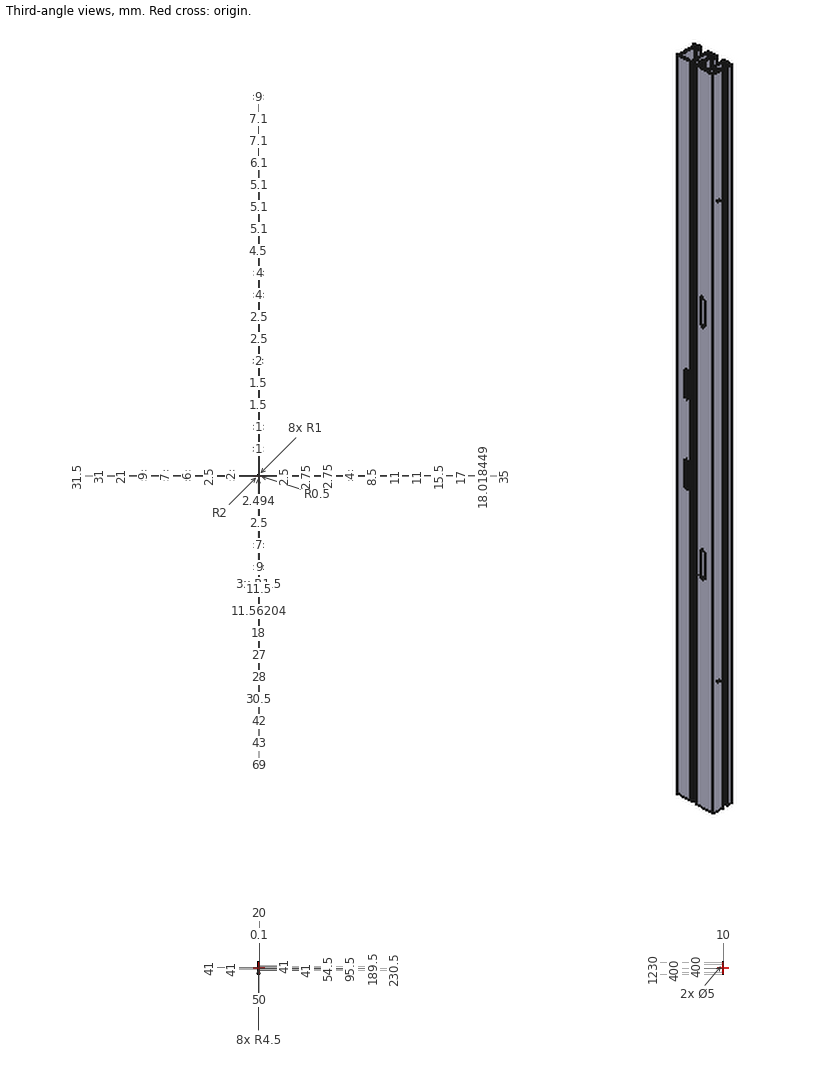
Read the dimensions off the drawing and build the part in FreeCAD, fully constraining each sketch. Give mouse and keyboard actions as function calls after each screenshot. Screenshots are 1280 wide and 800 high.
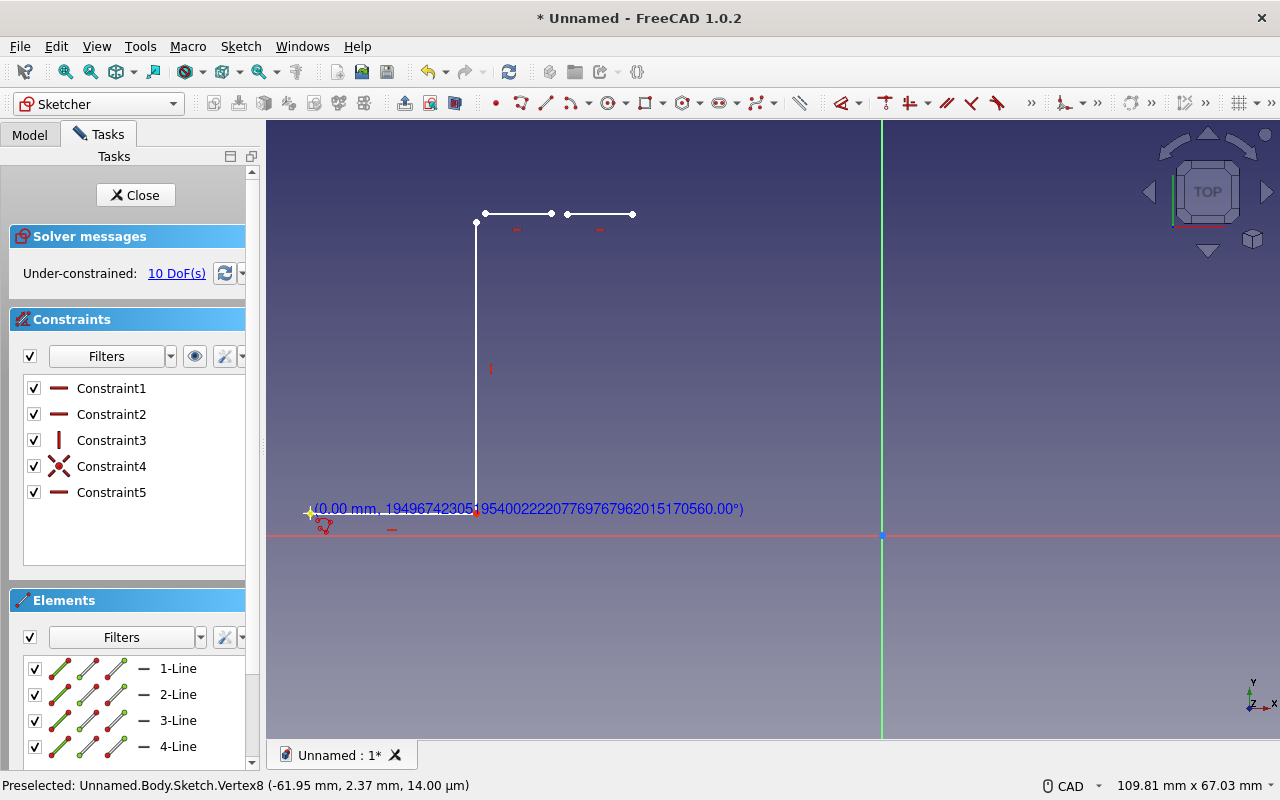
click(546, 104)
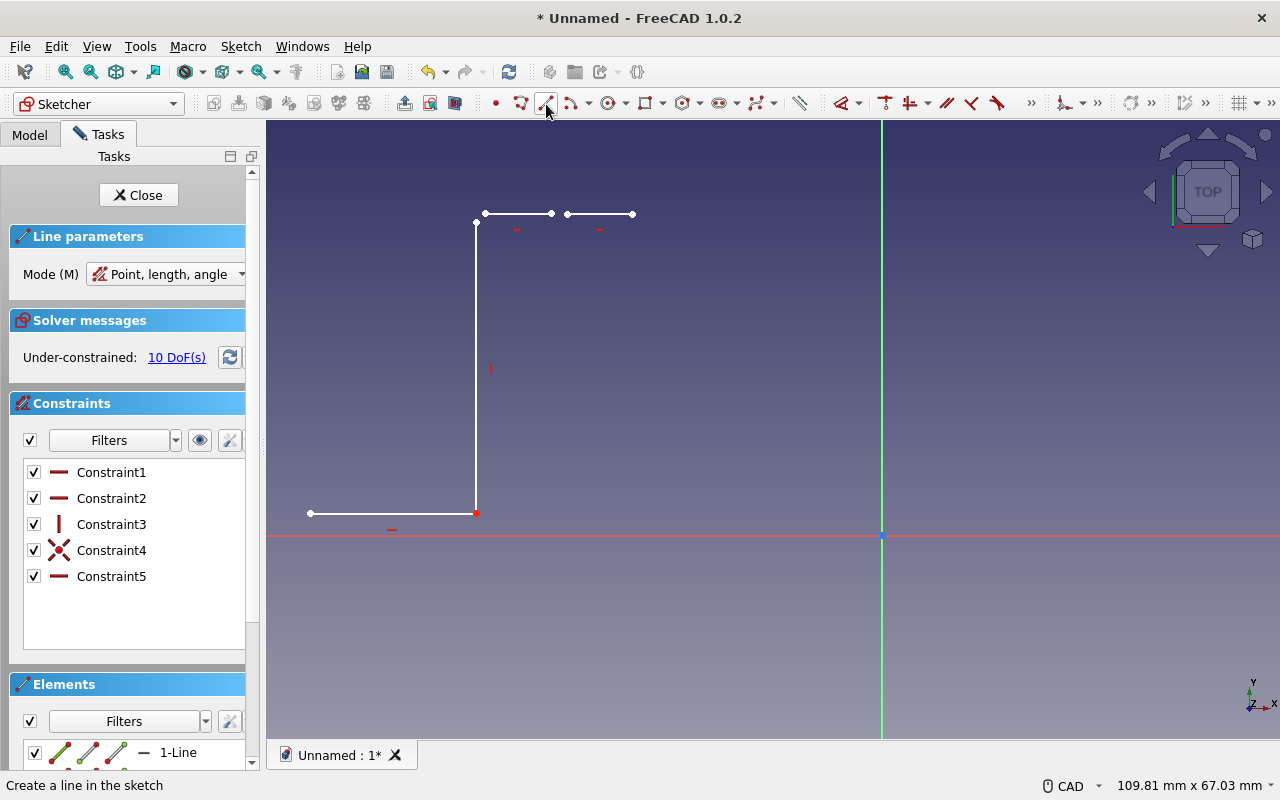
scroll(1115, 679, down, 1)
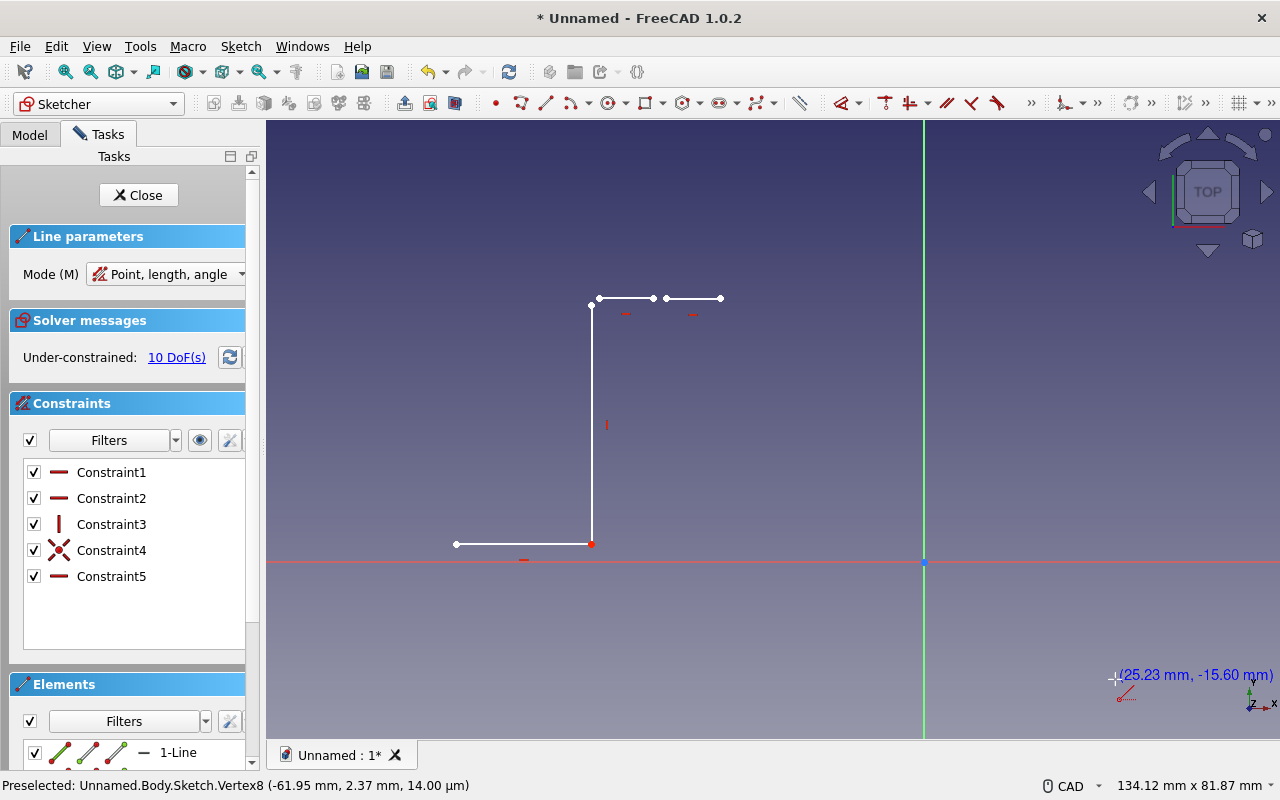
click(441, 528)
click(441, 328)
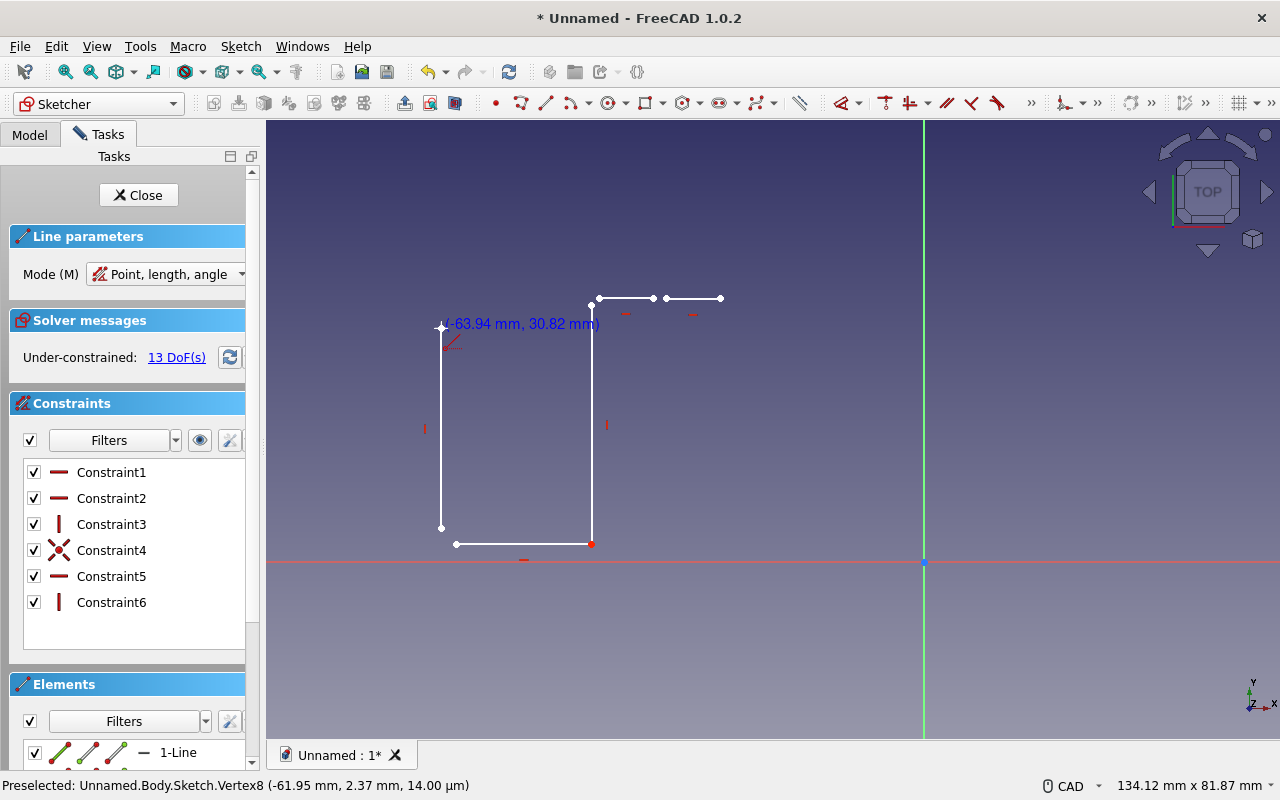
click(521, 104)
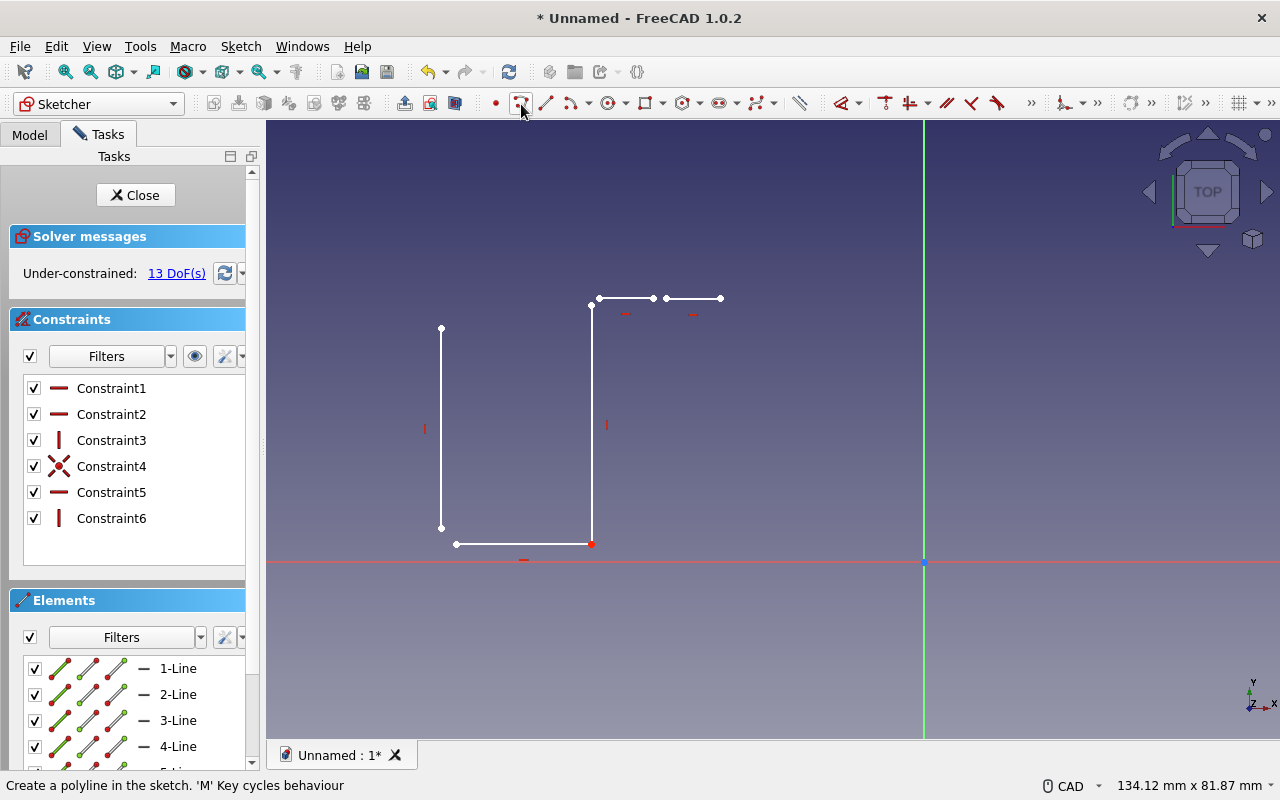
scroll(448, 320, up, 2)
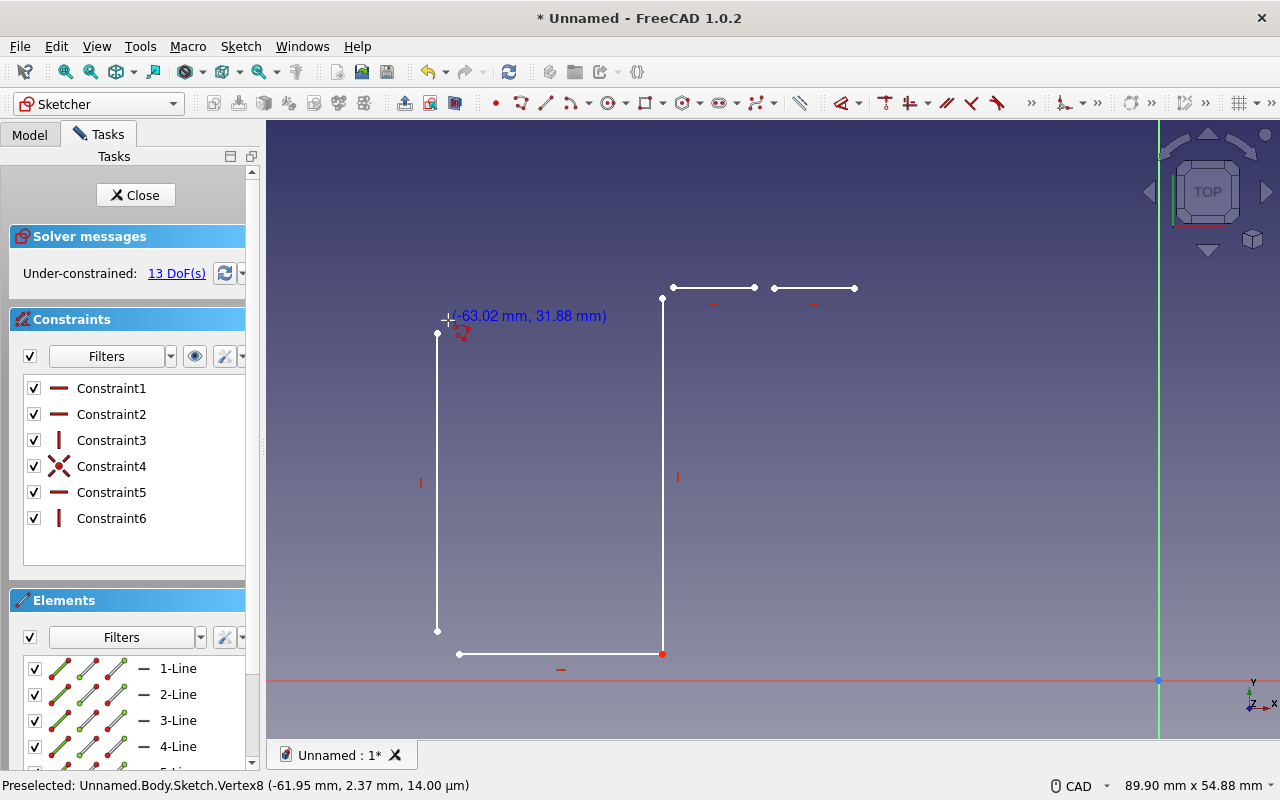
click(448, 320)
click(499, 320)
click(510, 399)
click(527, 399)
click(527, 297)
right_click(527, 297)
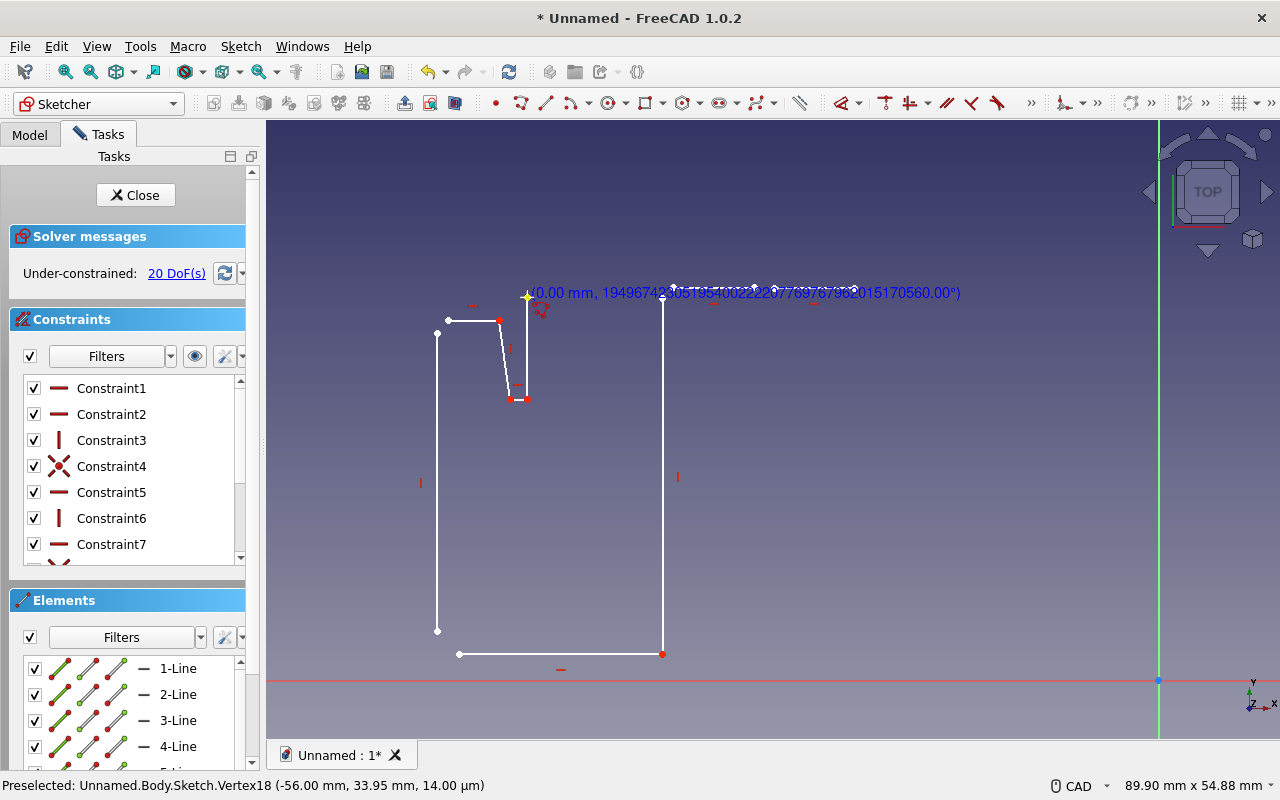
click(546, 104)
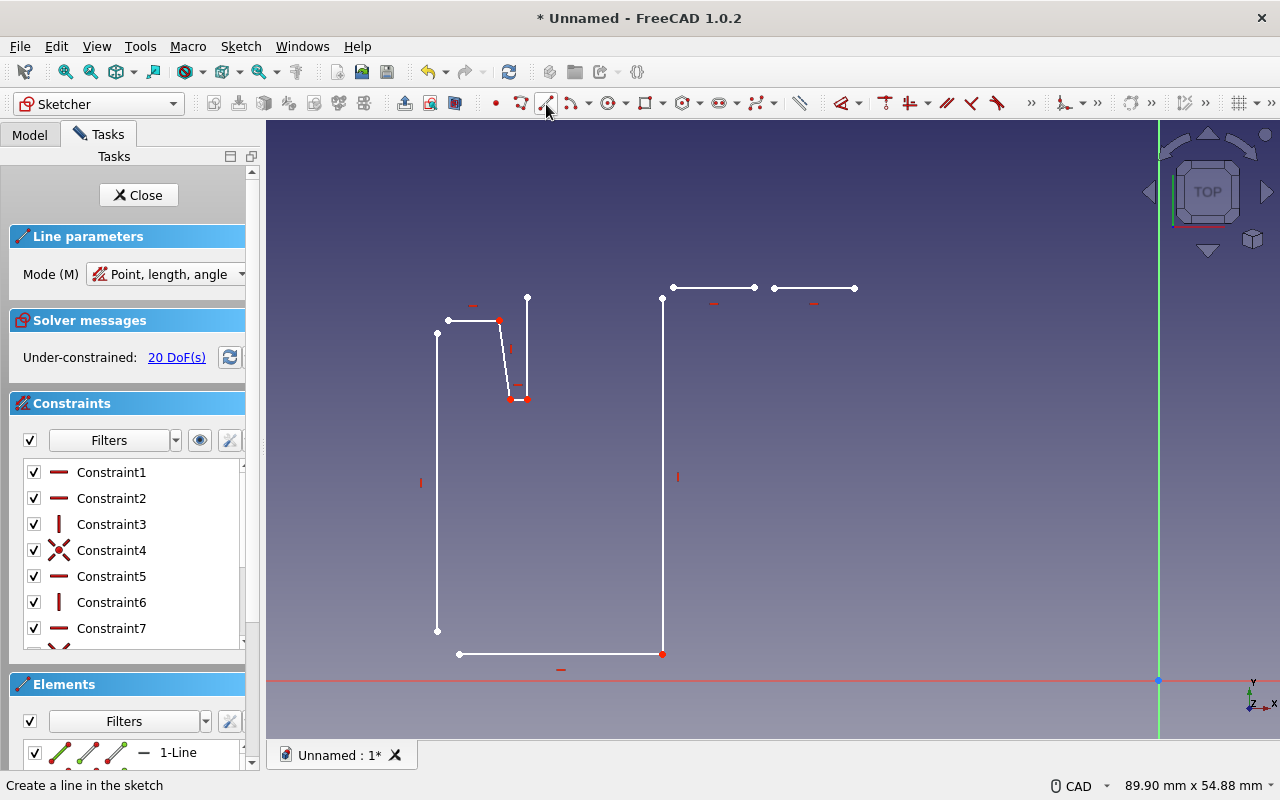
click(516, 286)
click(458, 286)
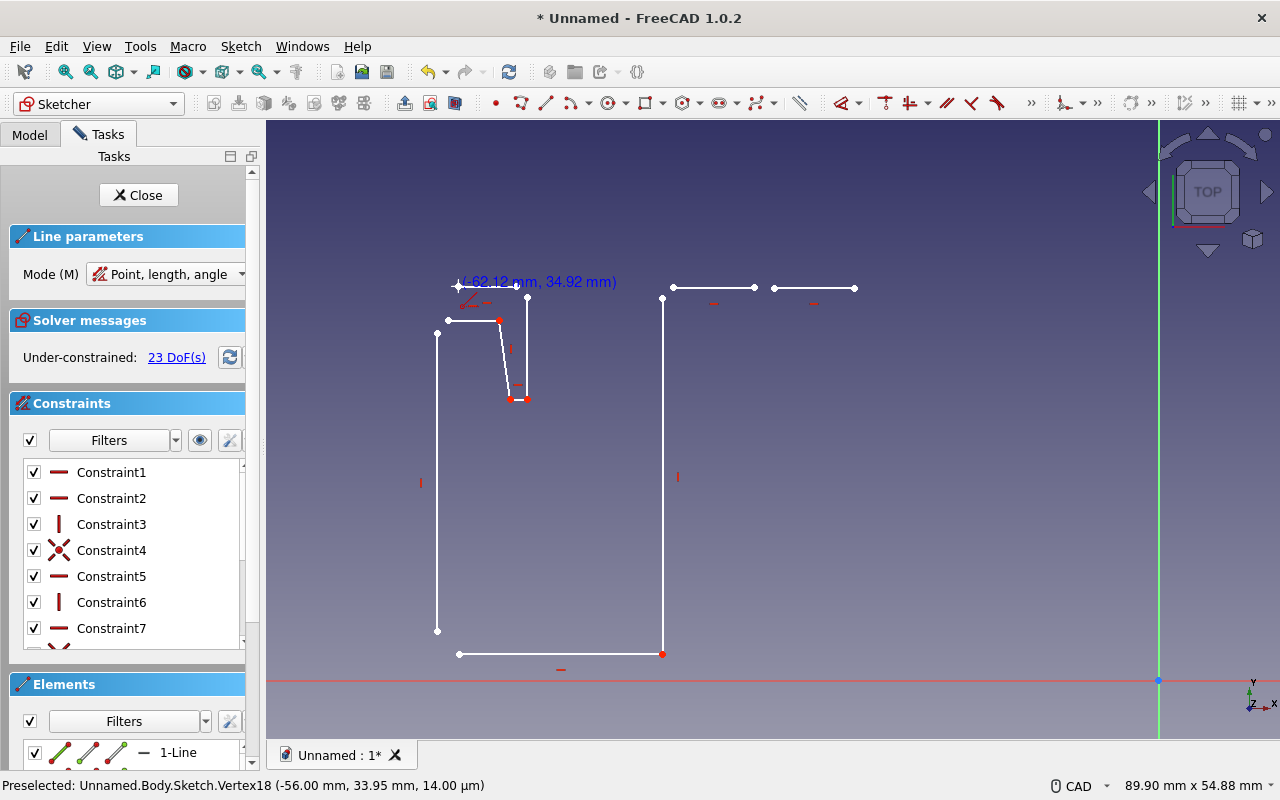
click(438, 286)
click(380, 286)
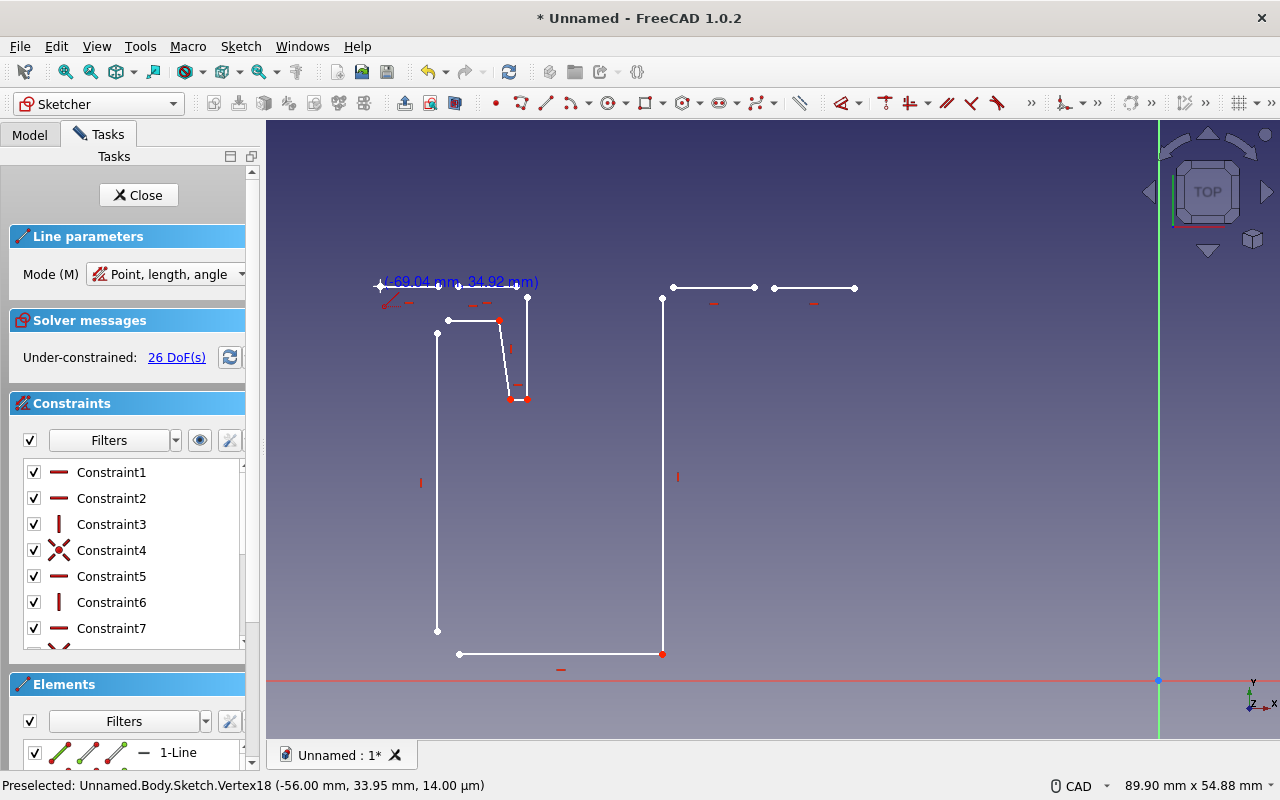
click(521, 104)